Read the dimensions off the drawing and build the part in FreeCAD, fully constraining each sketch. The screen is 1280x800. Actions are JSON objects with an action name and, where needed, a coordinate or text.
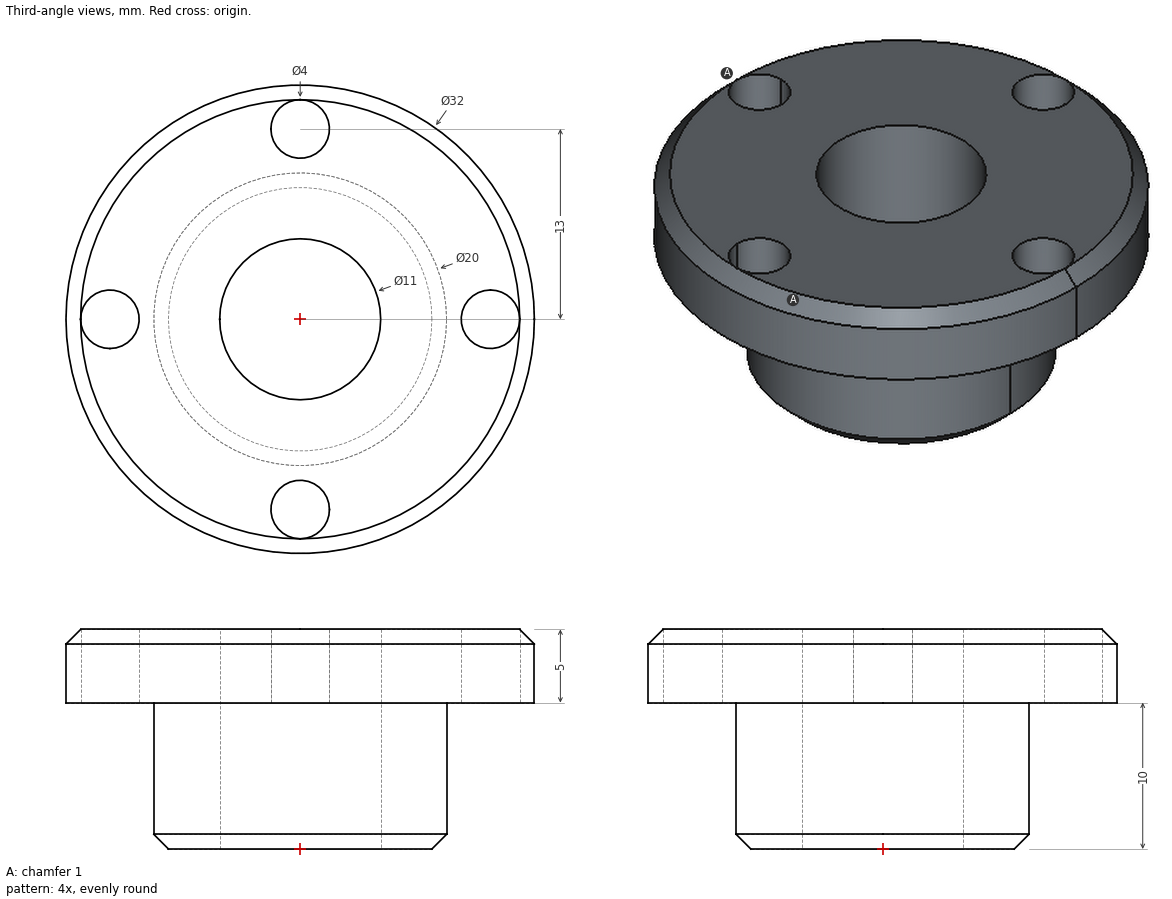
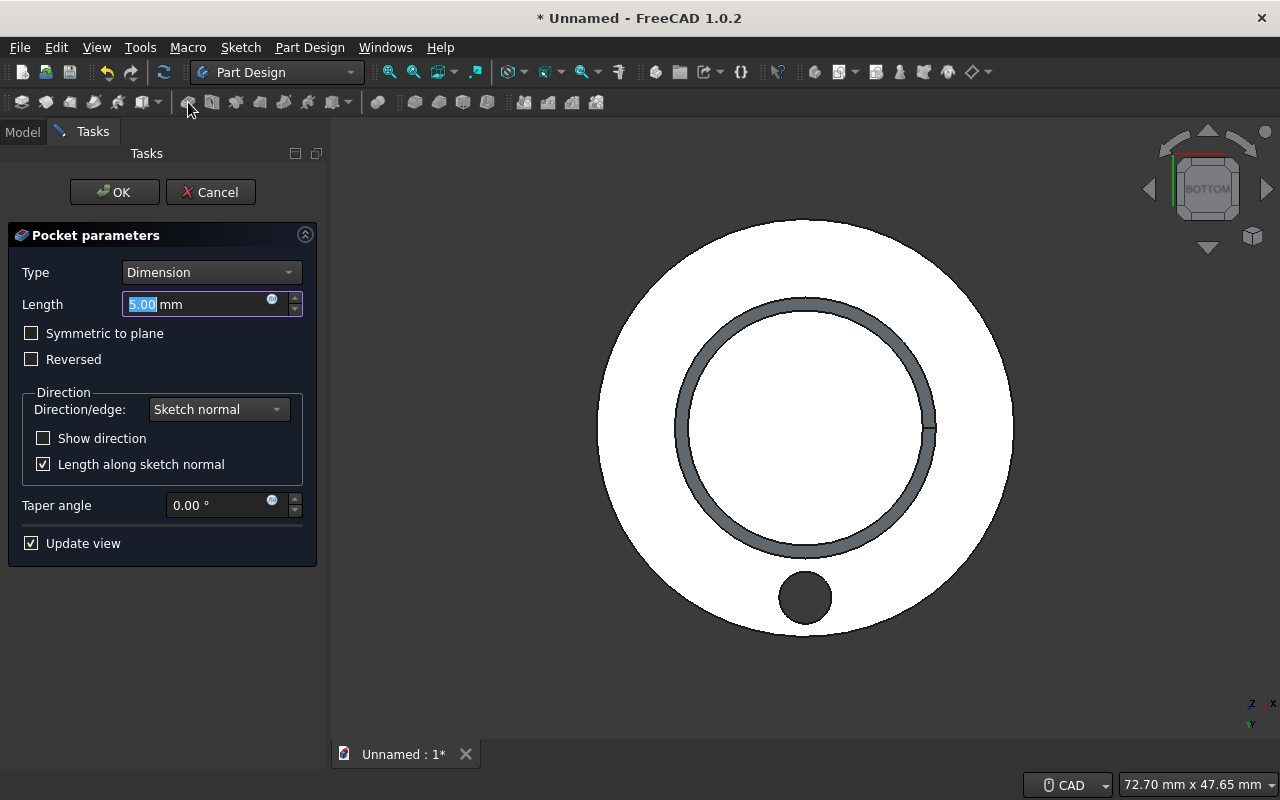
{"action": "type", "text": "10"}
{"action": "key", "text": "Tab"}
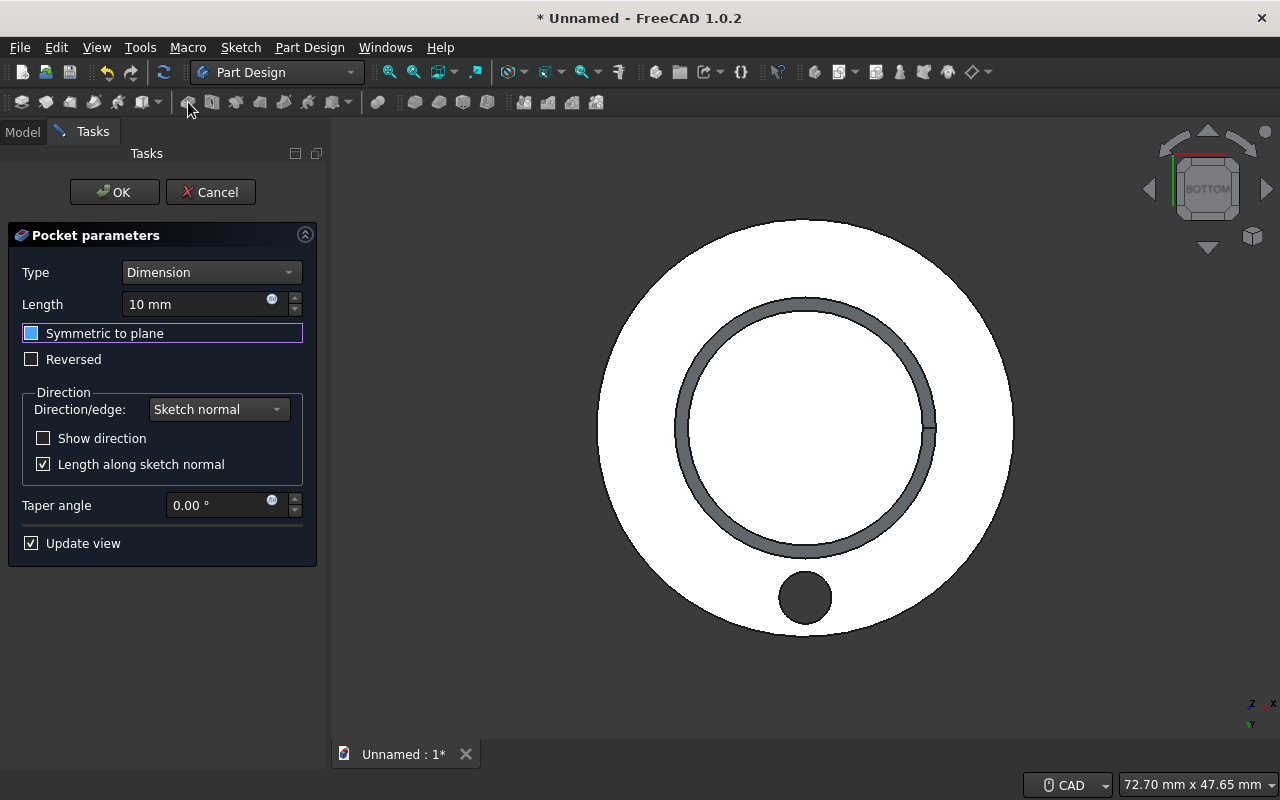
{"action": "left_click", "coordinate": [115, 192]}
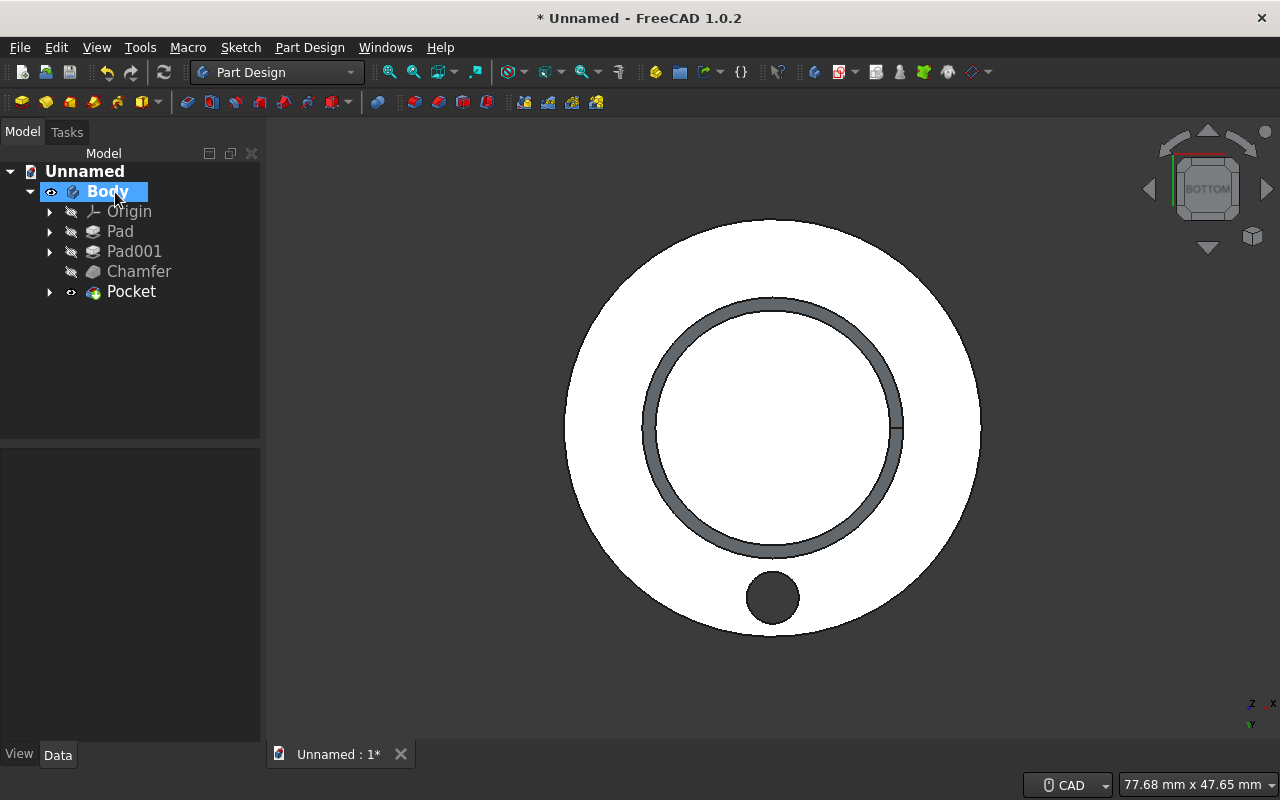
{"action": "left_click", "coordinate": [116, 292]}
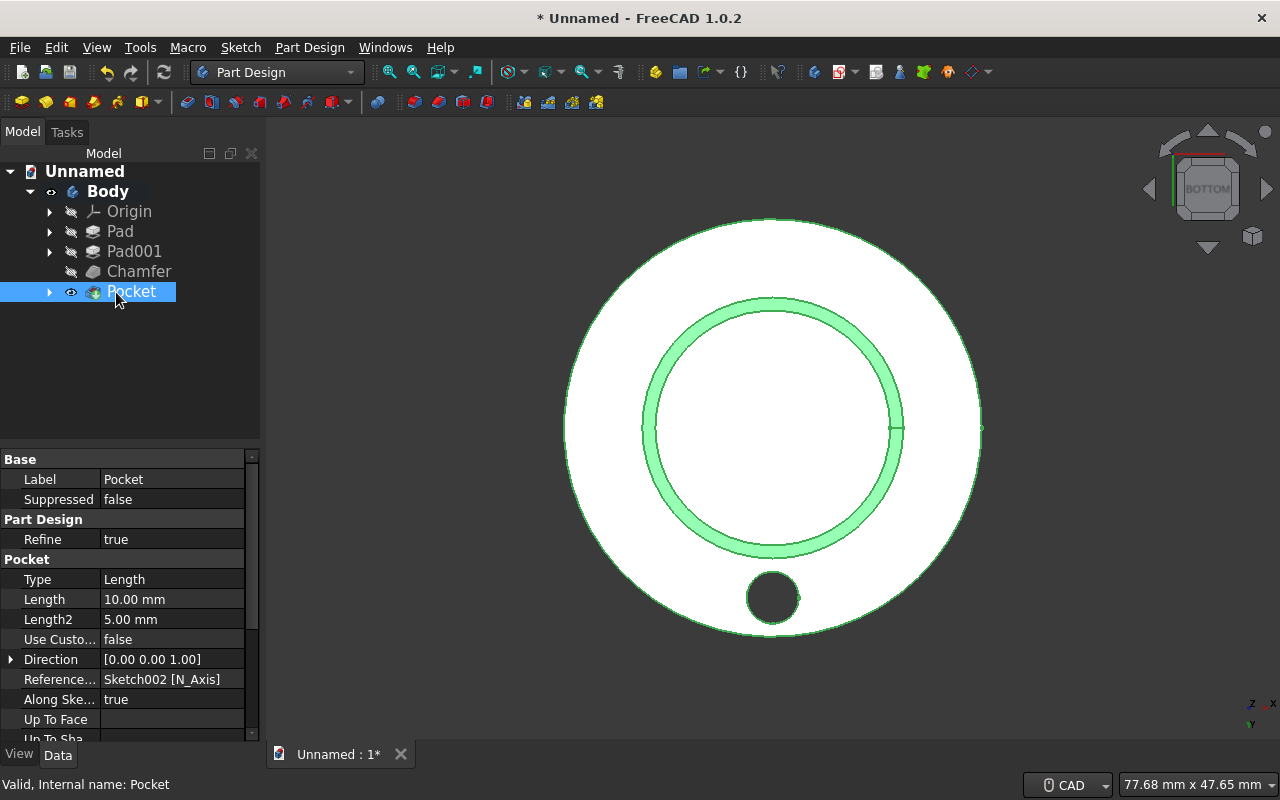
{"action": "left_click", "coordinate": [572, 102]}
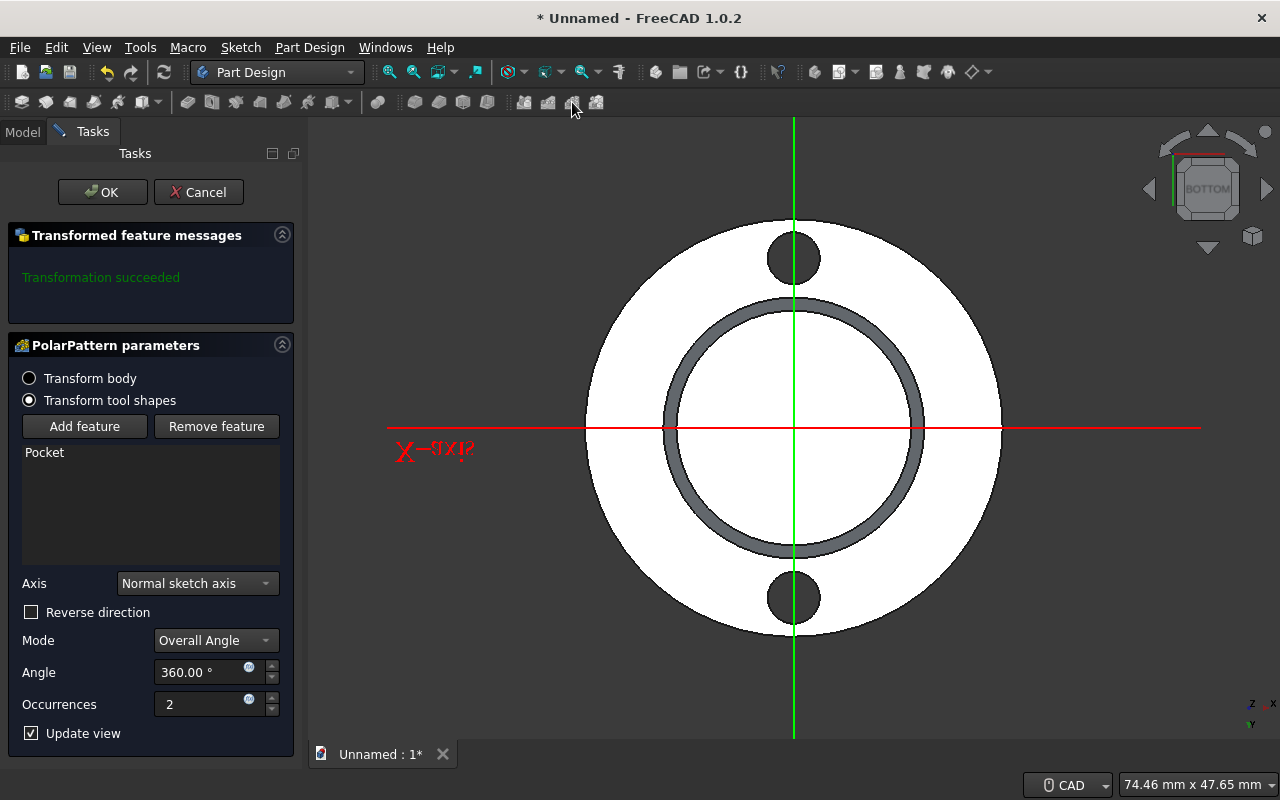
{"action": "left_click", "coordinate": [198, 584]}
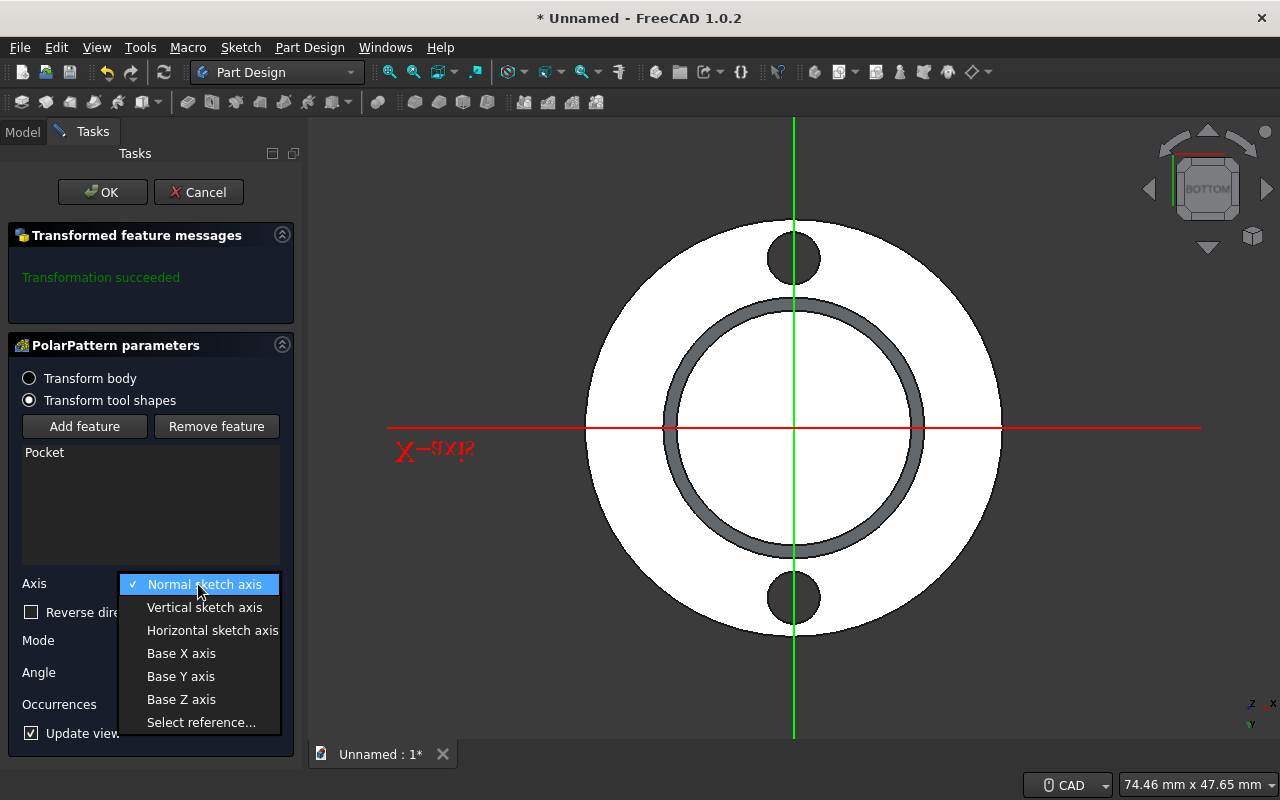
{"action": "left_click", "coordinate": [198, 700]}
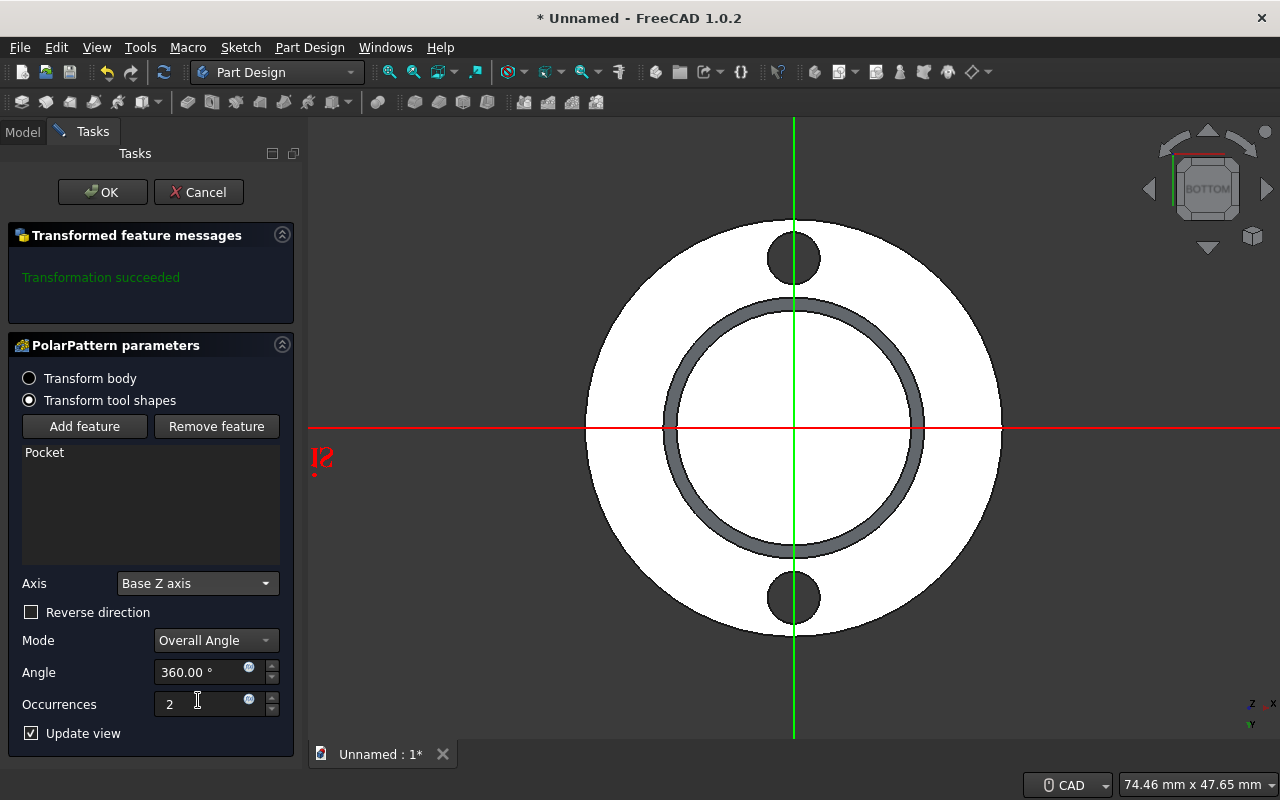
{"action": "triple_click", "coordinate": [209, 704]}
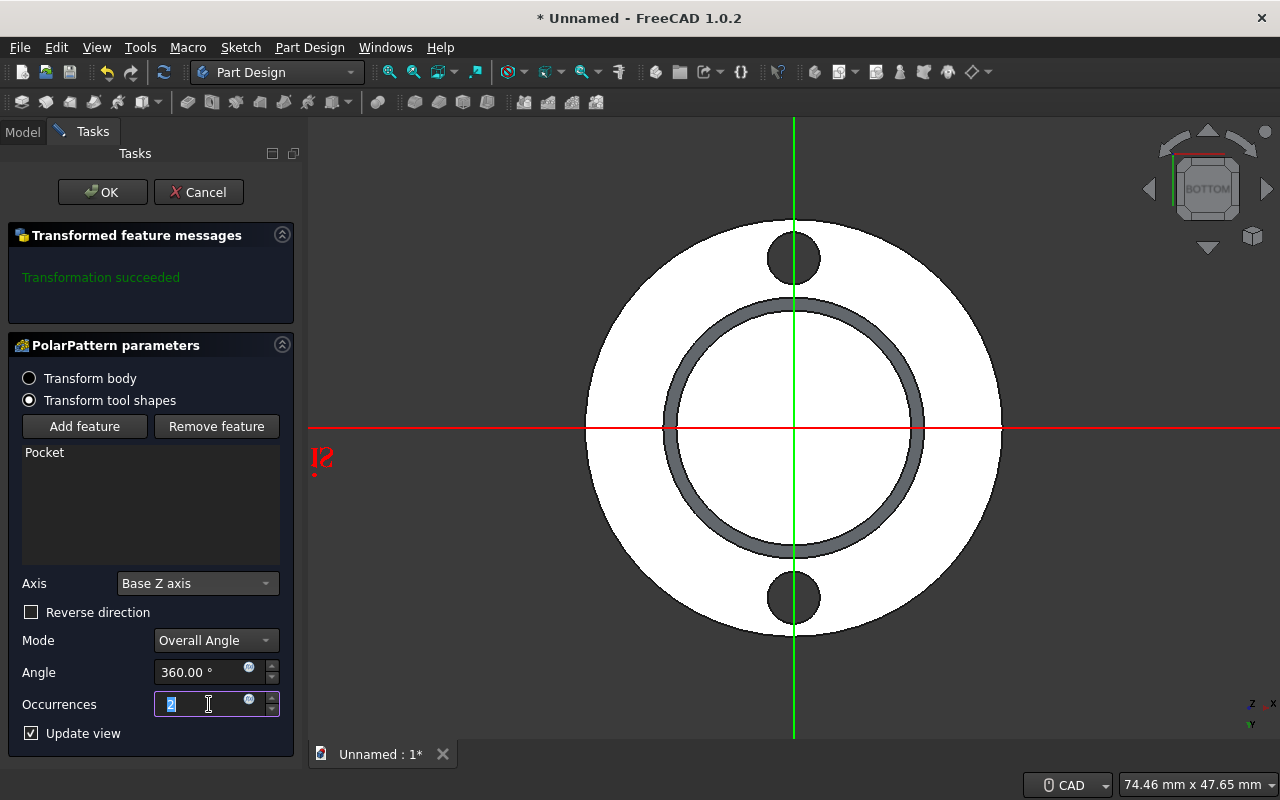
{"action": "type", "text": "4"}
{"action": "key", "text": "Tab"}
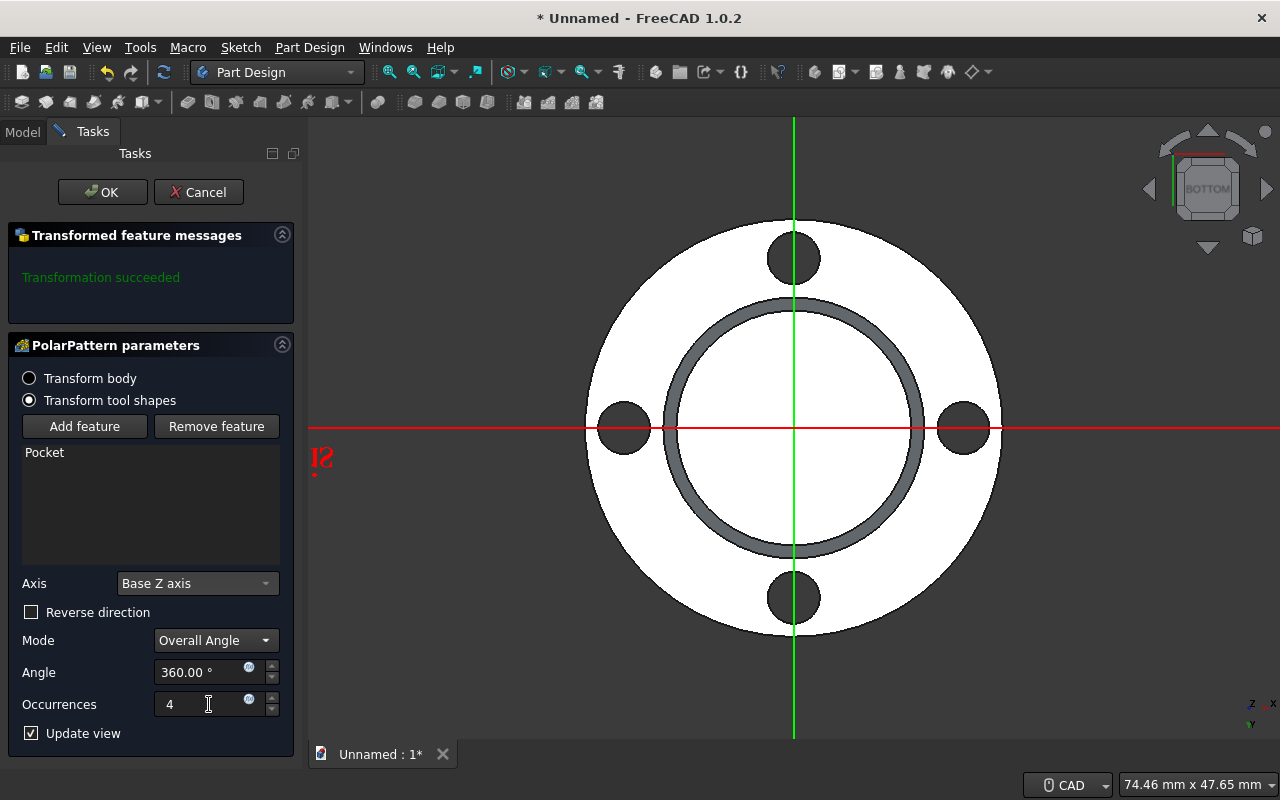
{"action": "left_click", "coordinate": [103, 192]}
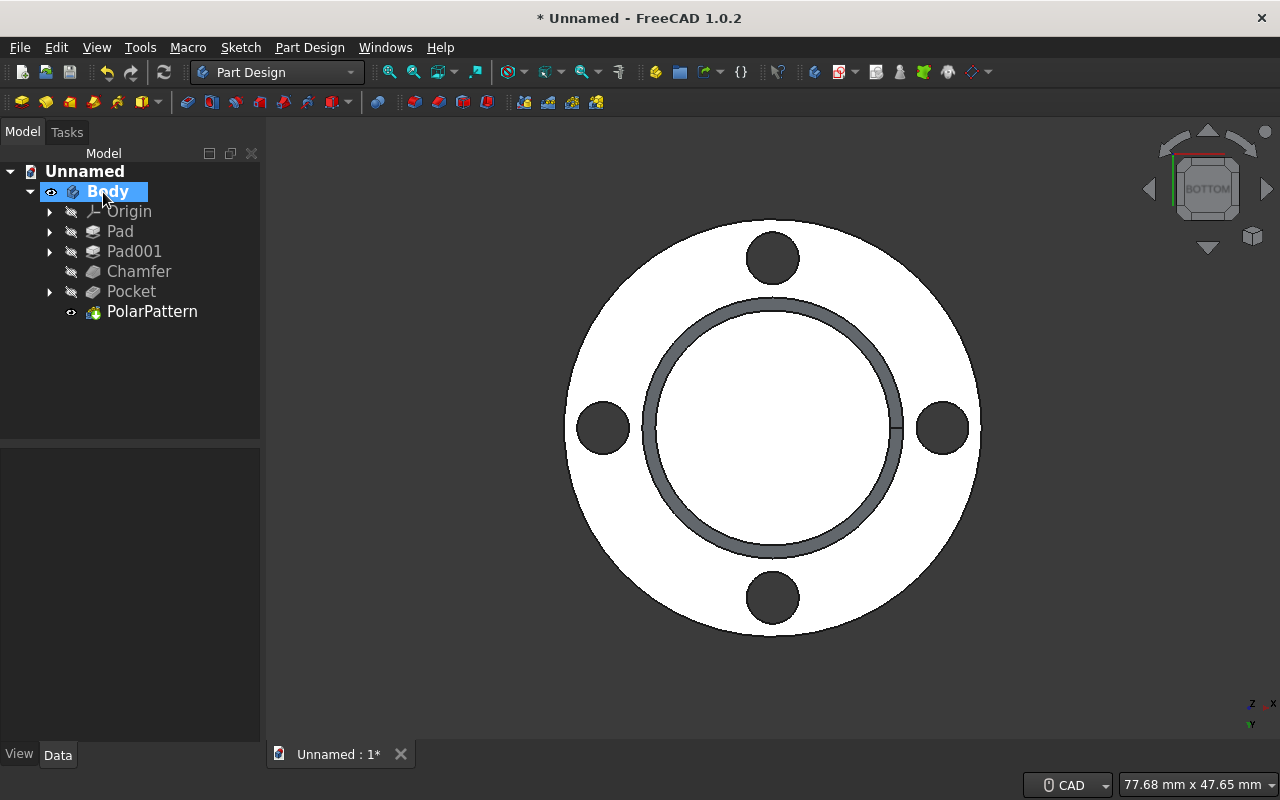
{"action": "left_click", "coordinate": [773, 427]}